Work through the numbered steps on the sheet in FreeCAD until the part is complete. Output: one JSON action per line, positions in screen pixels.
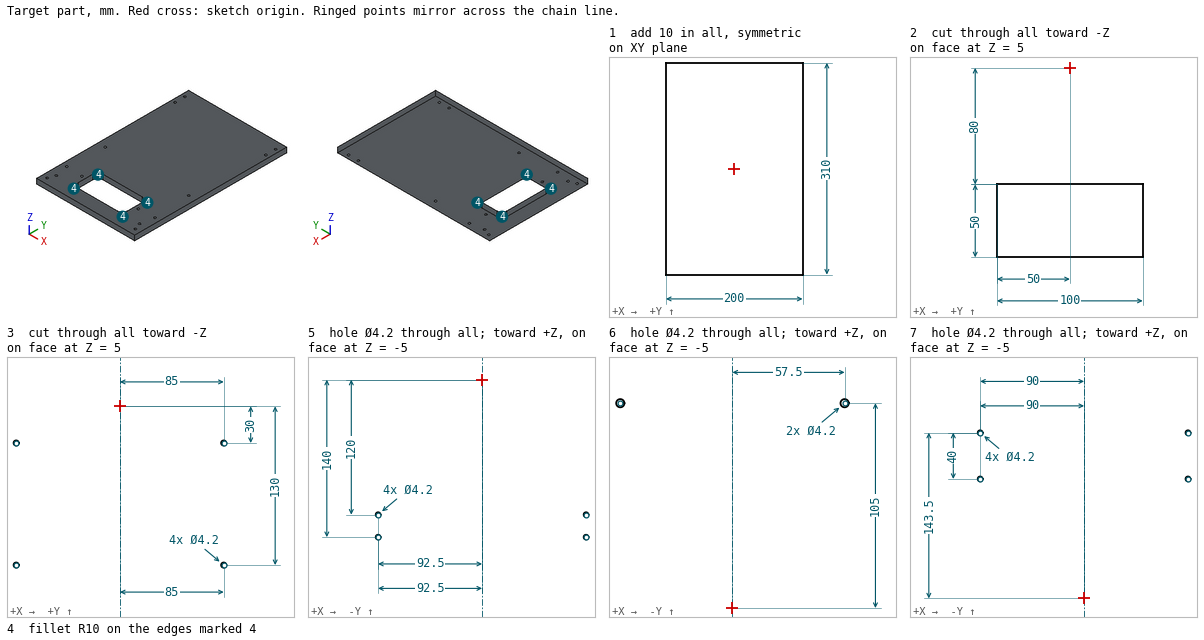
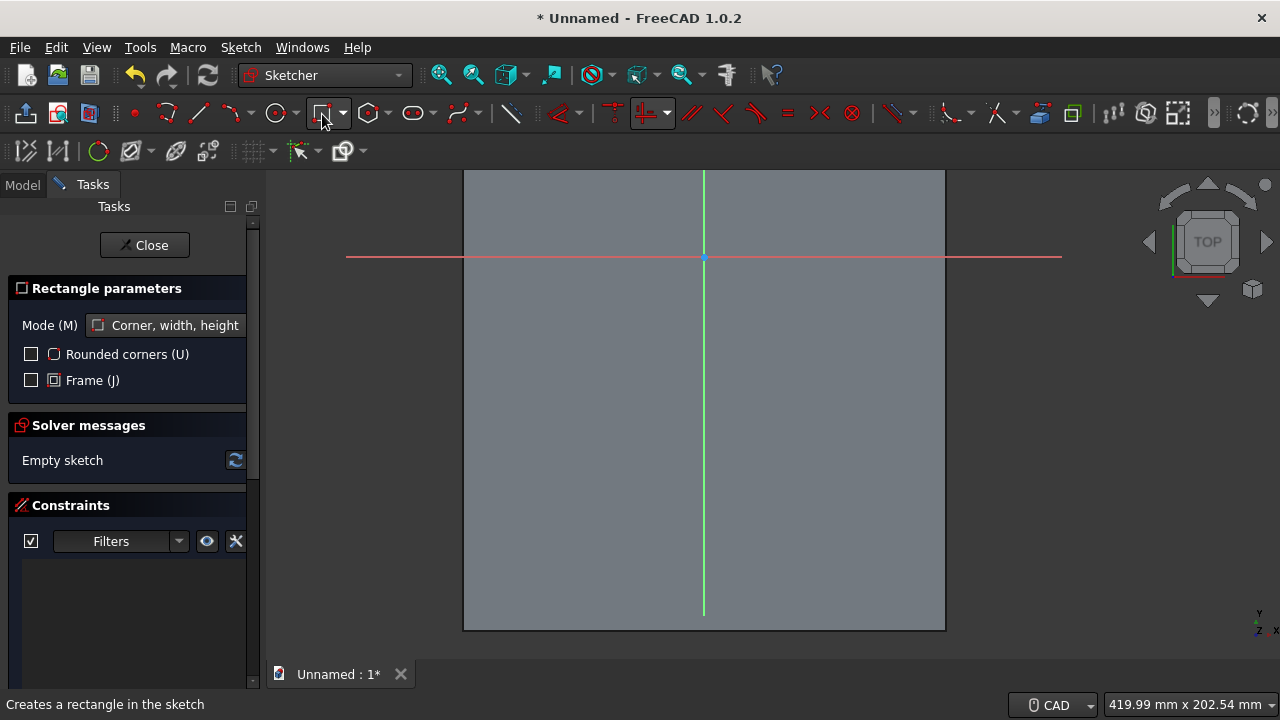
{"action": "left_click", "coordinate": [584, 450]}
{"action": "left_click", "coordinate": [825, 571]}
{"action": "key", "text": "Escape"}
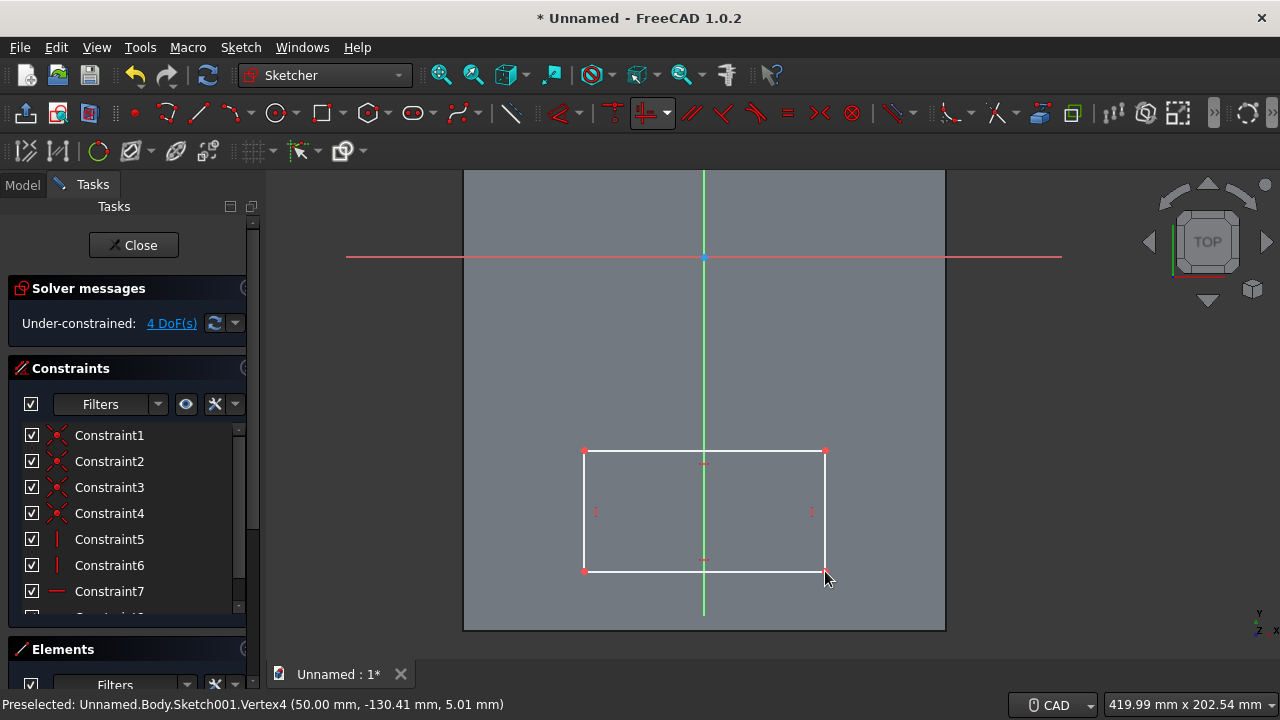
{"action": "key", "text": "d"}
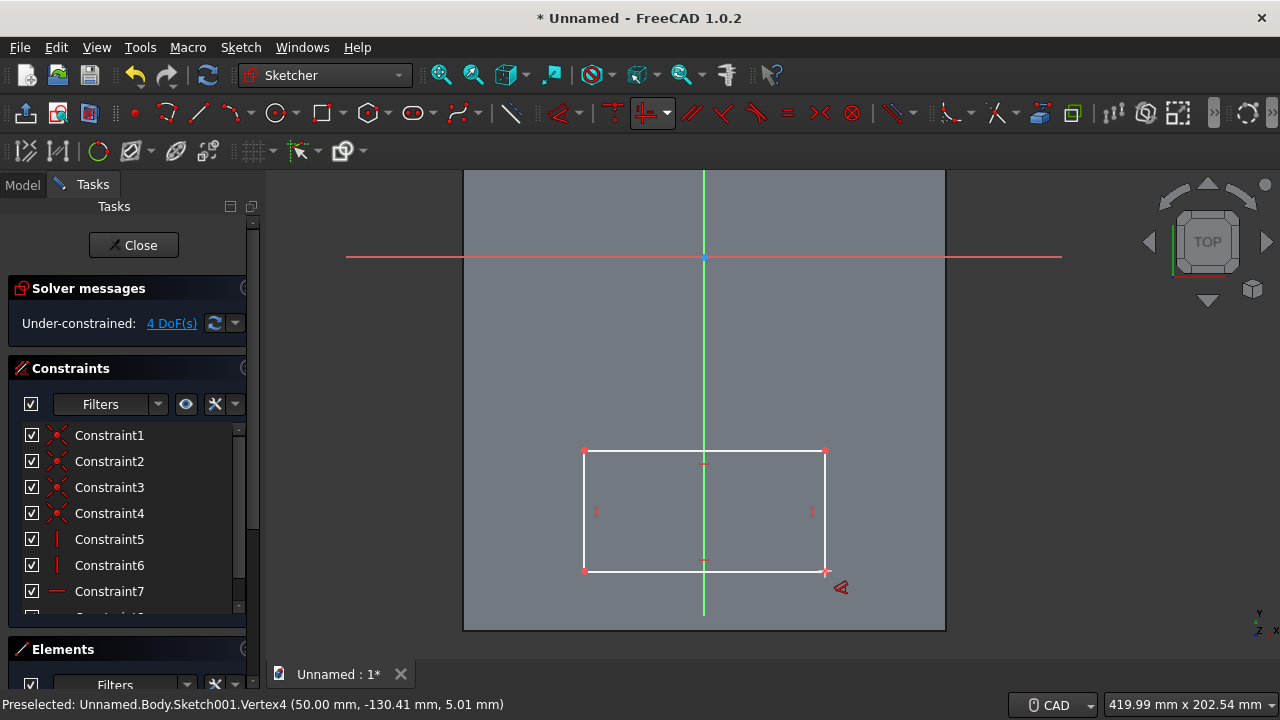
{"action": "left_click", "coordinate": [584, 487]}
{"action": "left_click", "coordinate": [550, 511]}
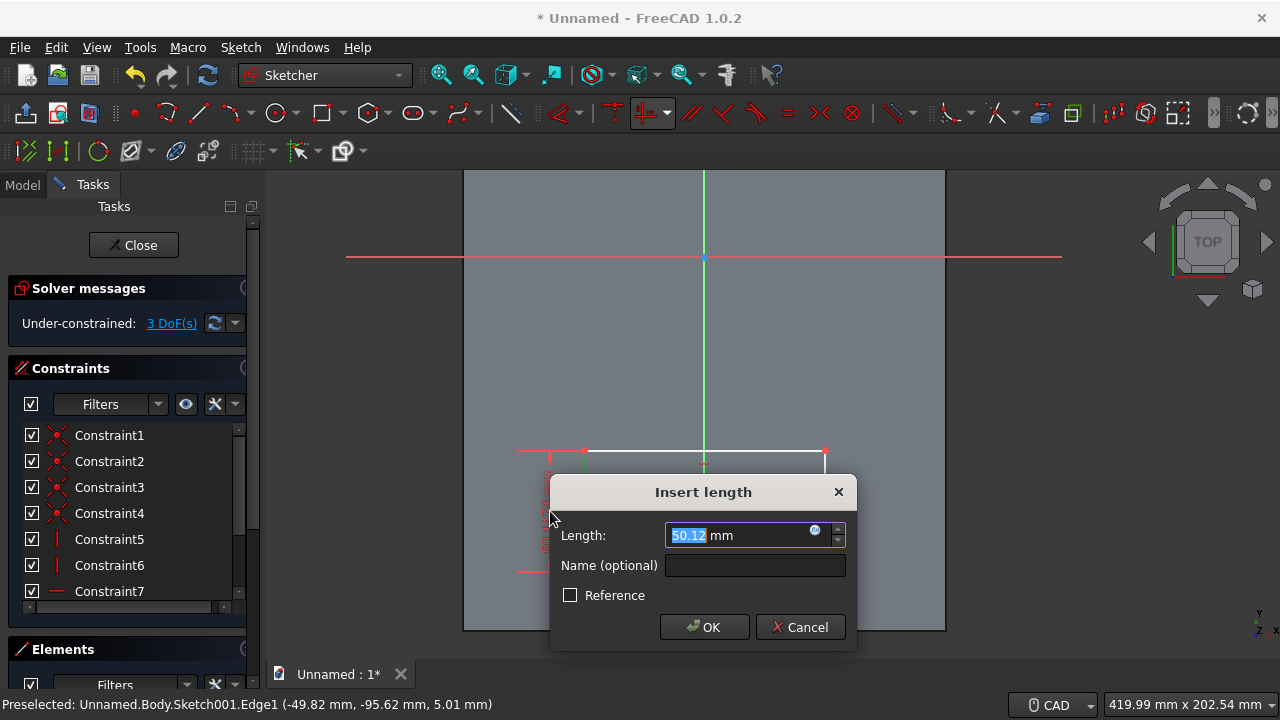
{"action": "type", "text": "50"}
{"action": "key", "text": "Return"}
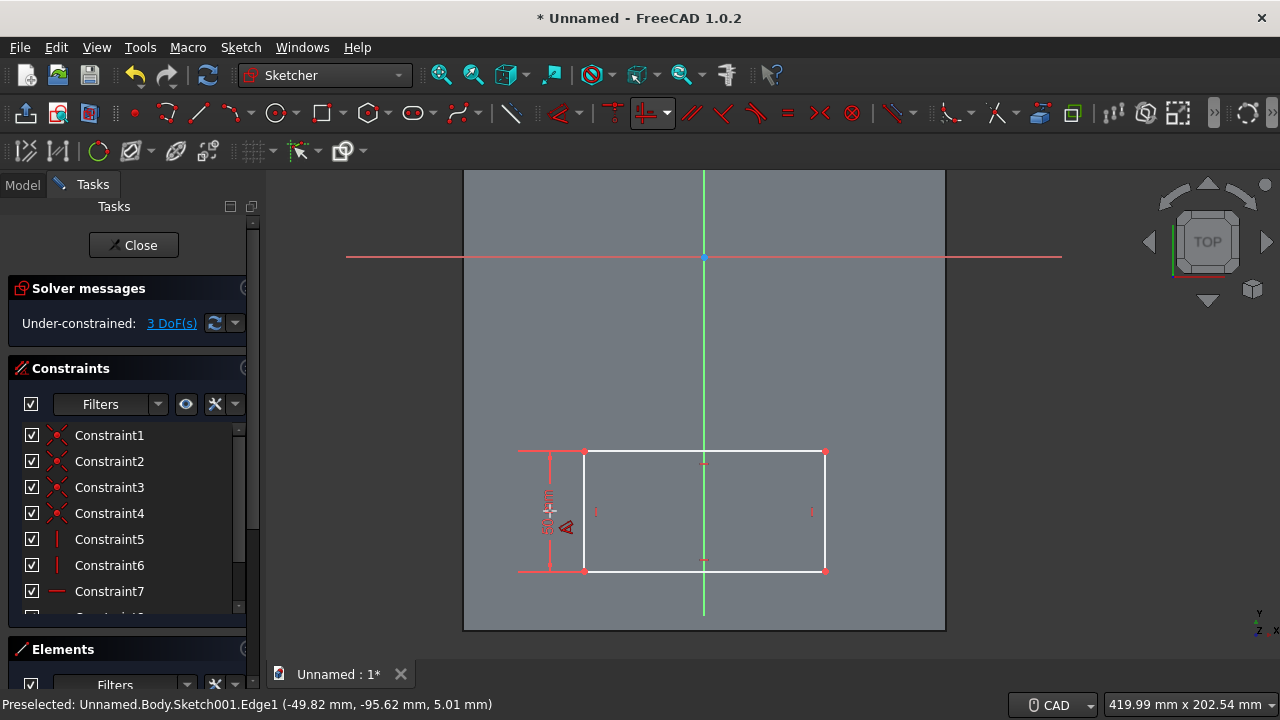
{"action": "left_click", "coordinate": [656, 572]}
{"action": "left_click", "coordinate": [649, 606]}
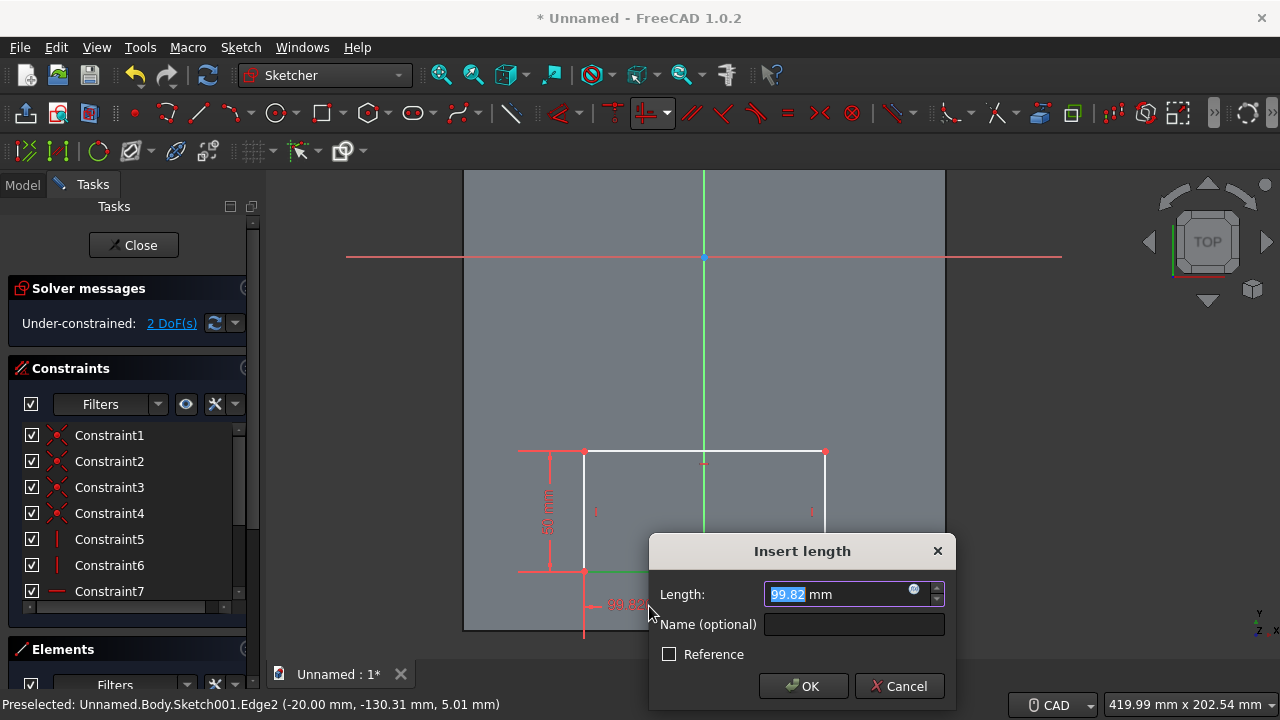
{"action": "type", "text": "100"}
{"action": "key", "text": "Return"}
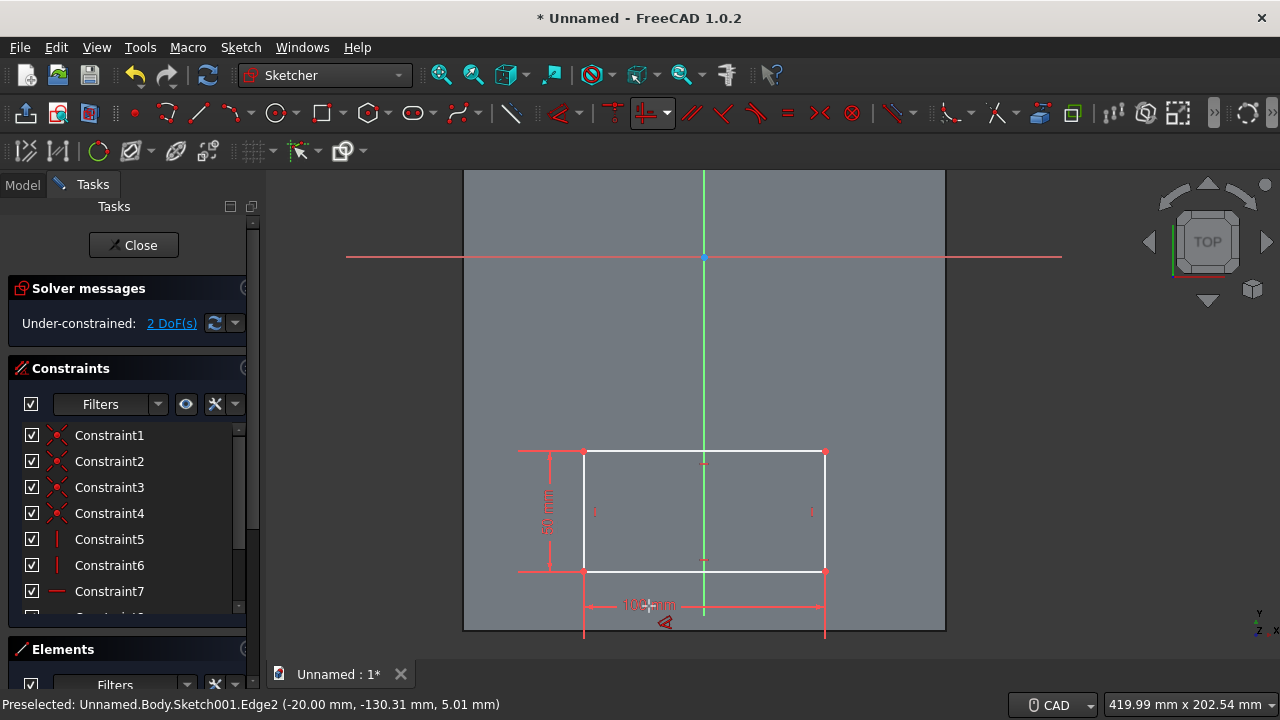
{"action": "left_click", "coordinate": [584, 451]}
{"action": "left_click", "coordinate": [644, 223]}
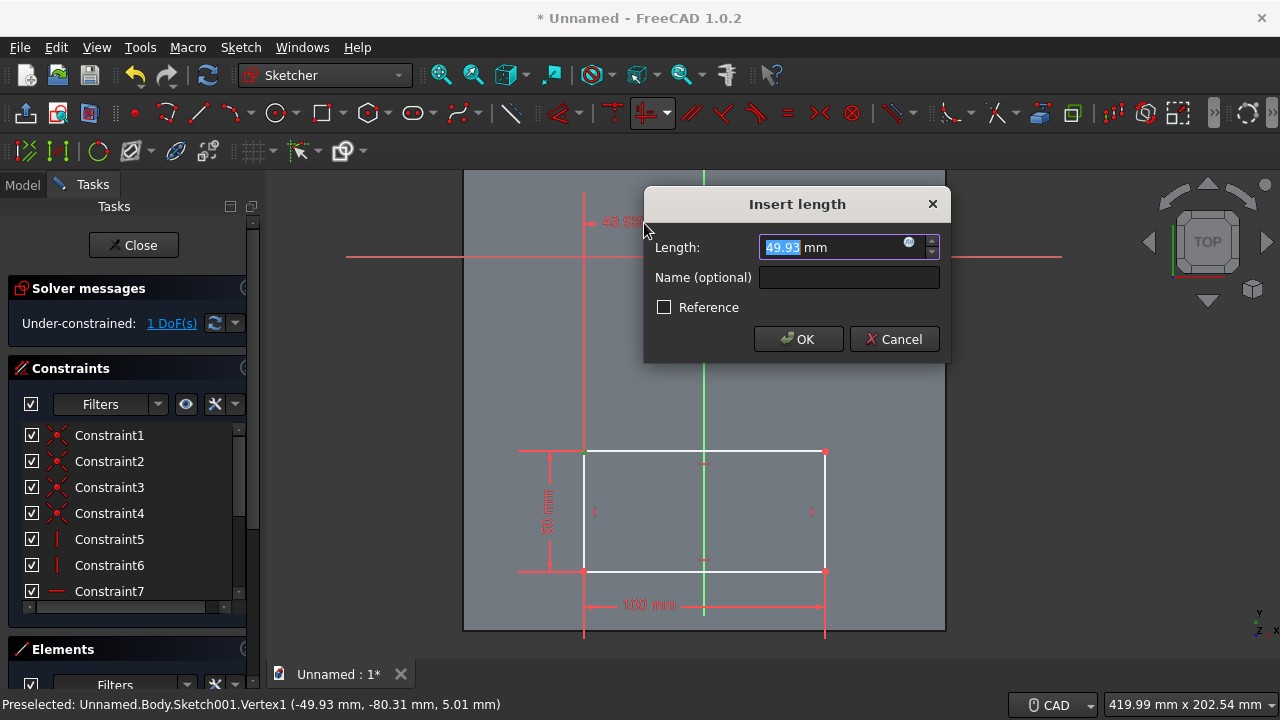
{"action": "type", "text": "50"}
{"action": "key", "text": "Return"}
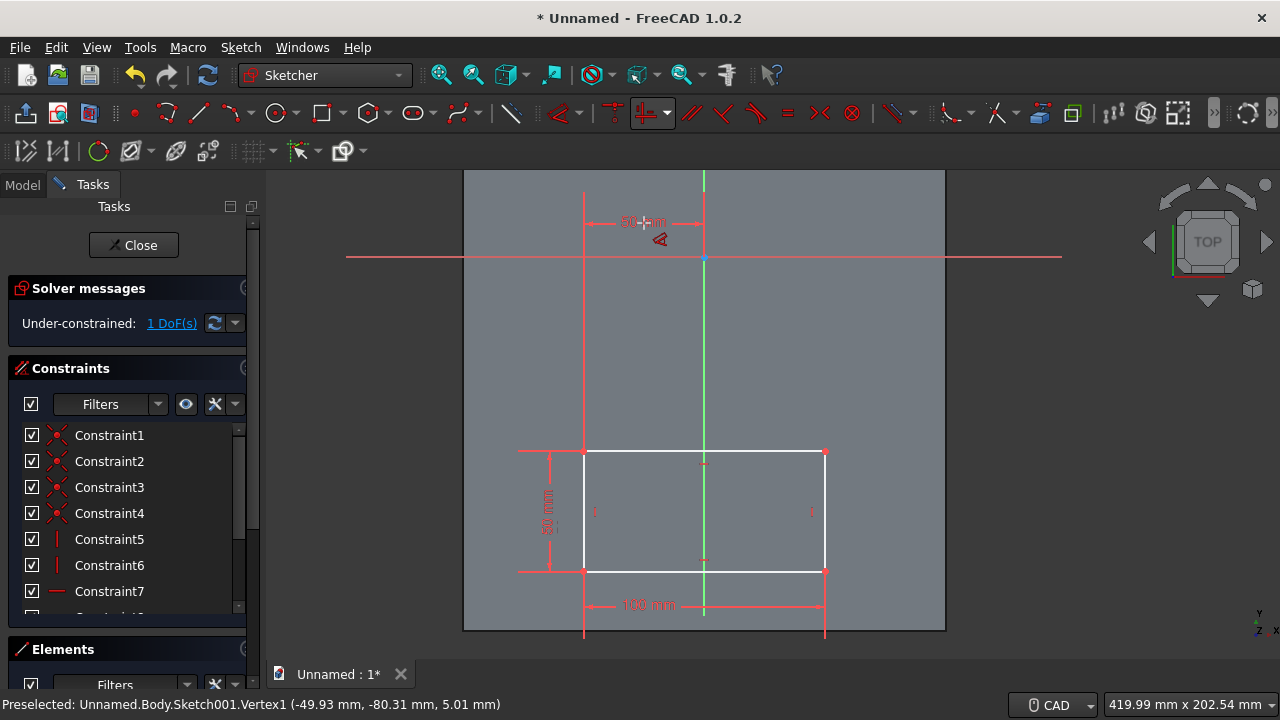
{"action": "left_click", "coordinate": [584, 451]}
{"action": "left_click", "coordinate": [550, 354]}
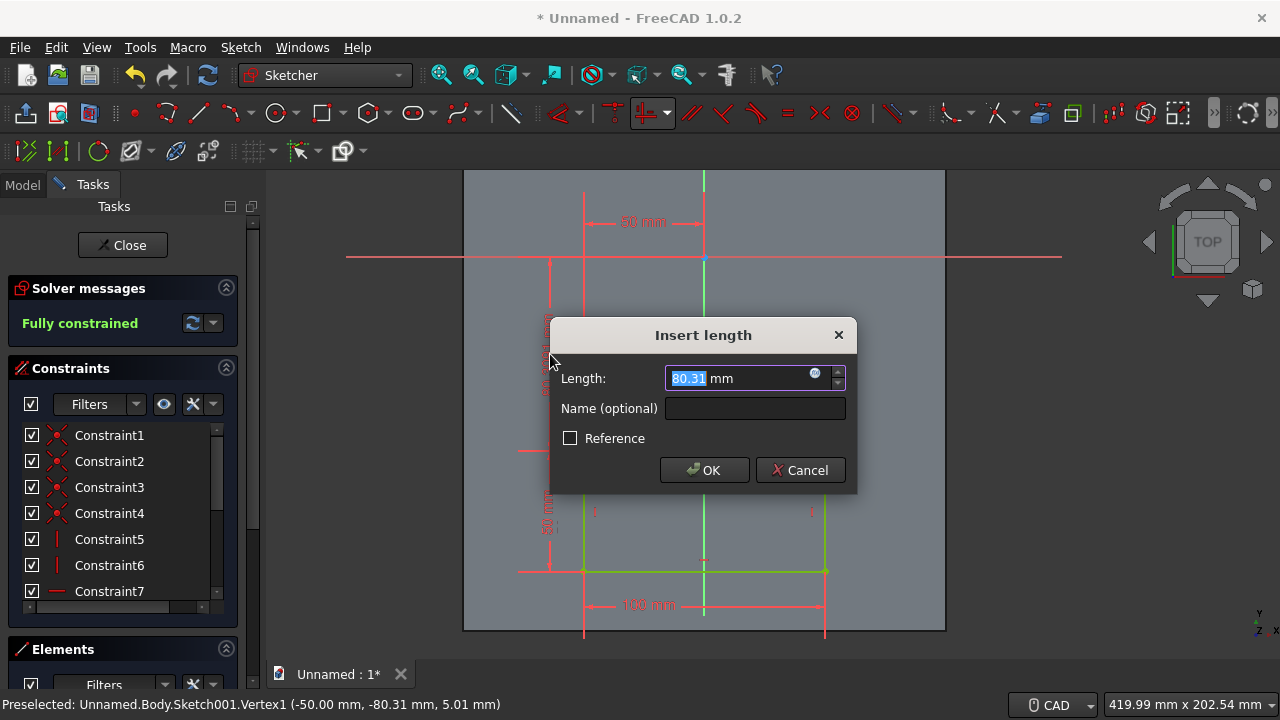
{"action": "type", "text": "80"}
{"action": "key", "text": "Return"}
{"action": "key", "text": "Escape"}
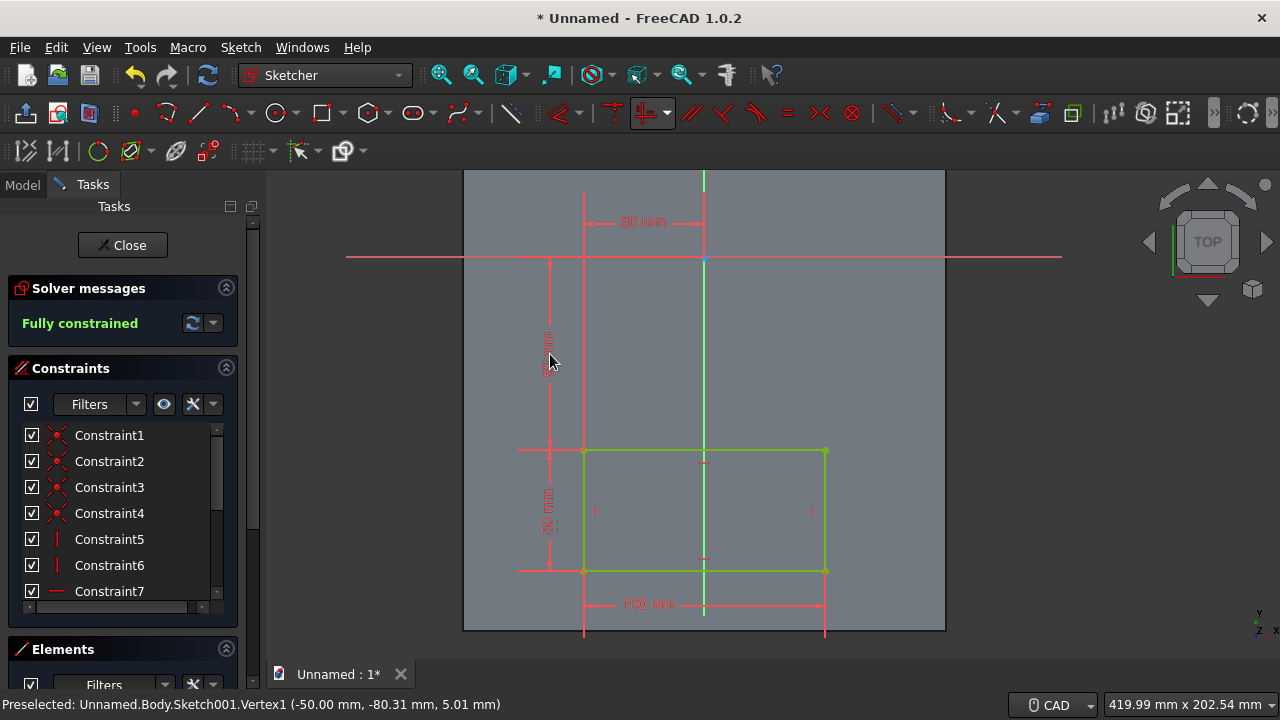
{"action": "left_click", "coordinate": [123, 245]}